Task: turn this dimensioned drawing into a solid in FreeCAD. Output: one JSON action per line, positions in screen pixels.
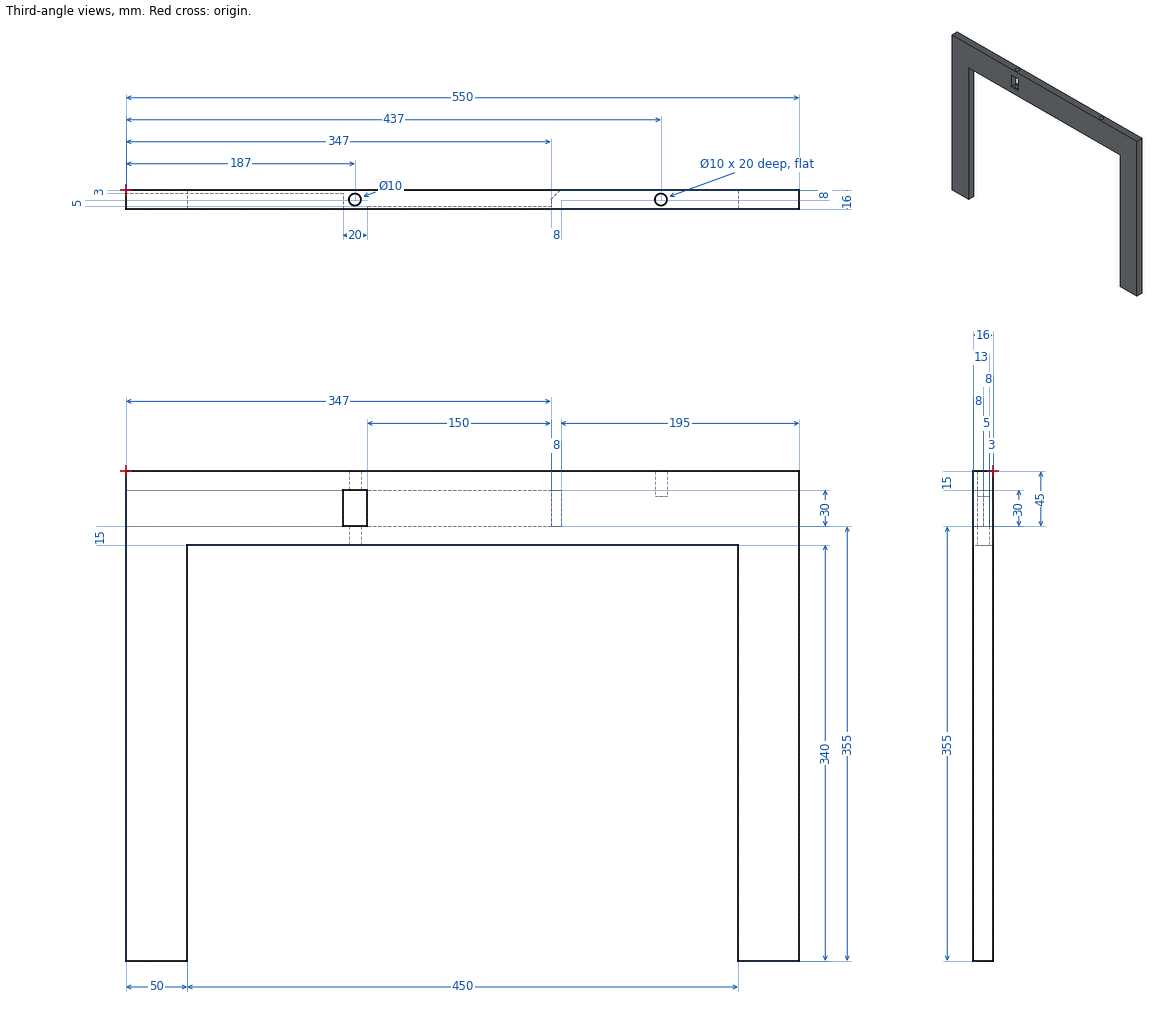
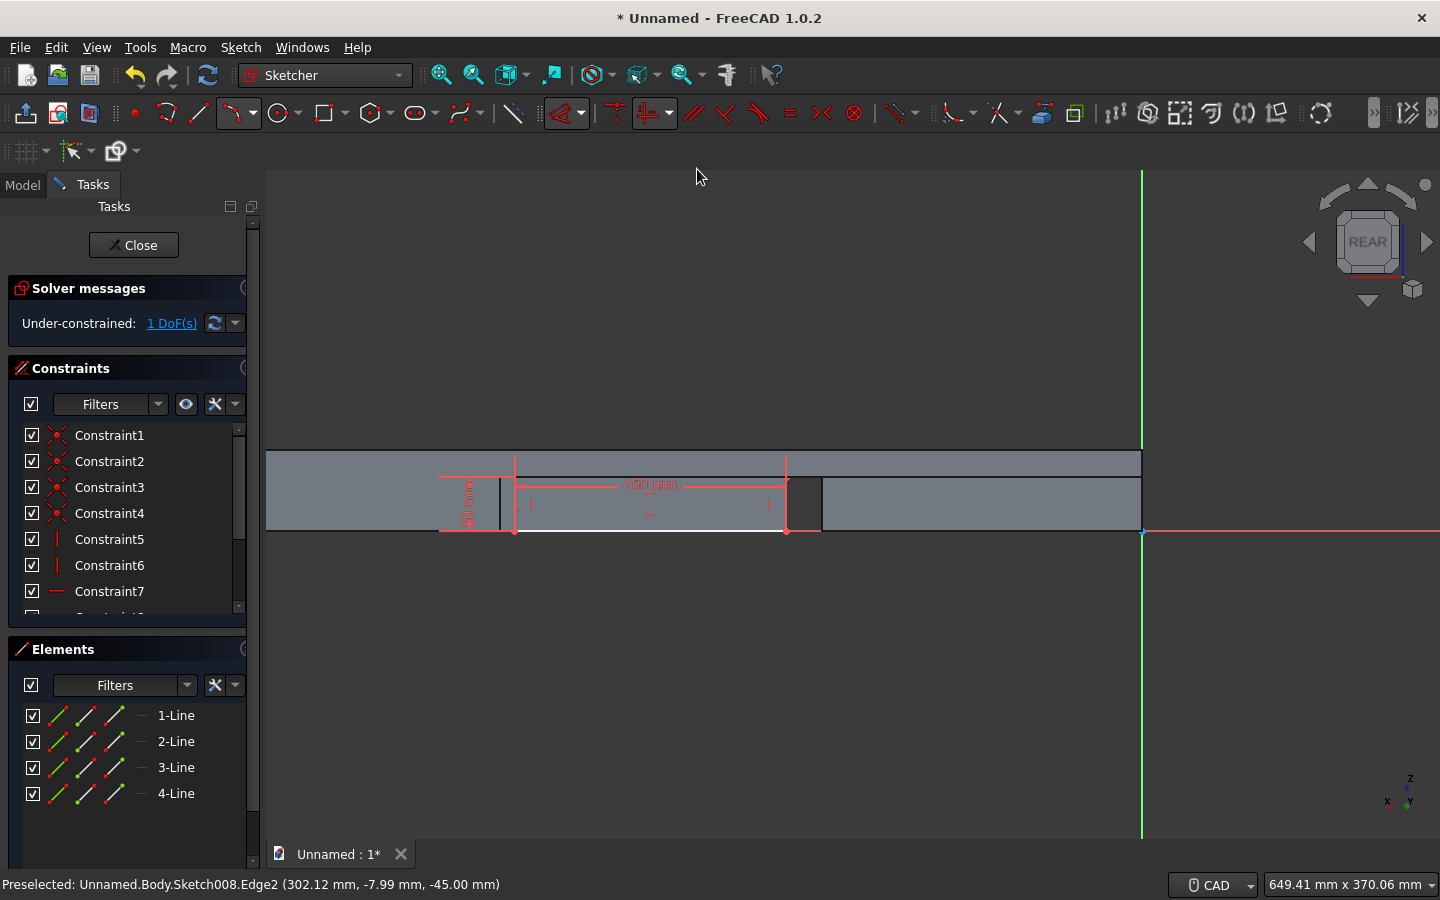
{"action": "left_click", "coordinate": [515, 477]}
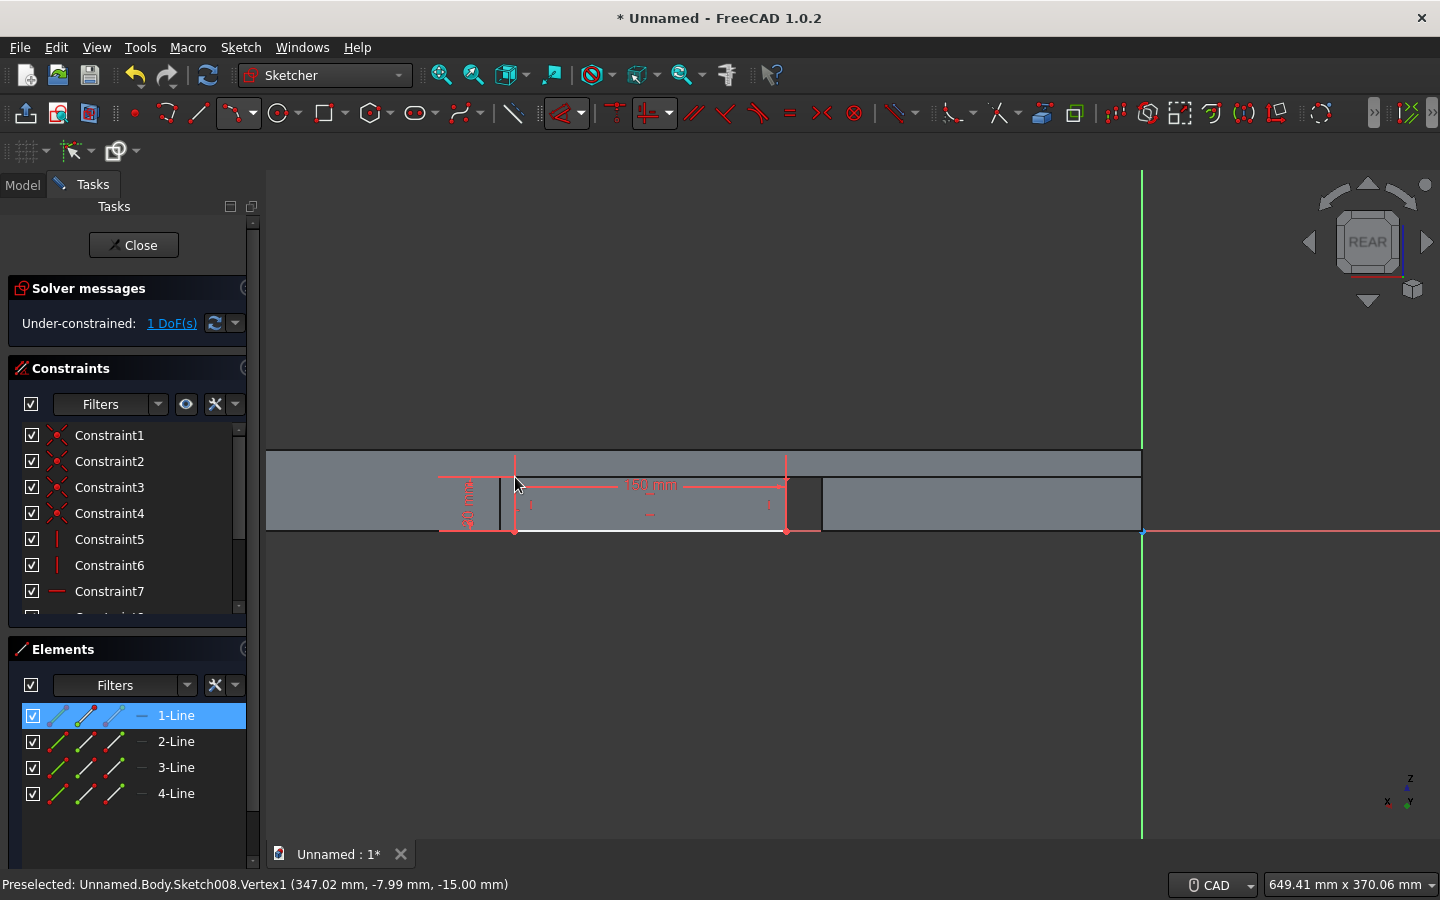
{"action": "key", "text": "l"}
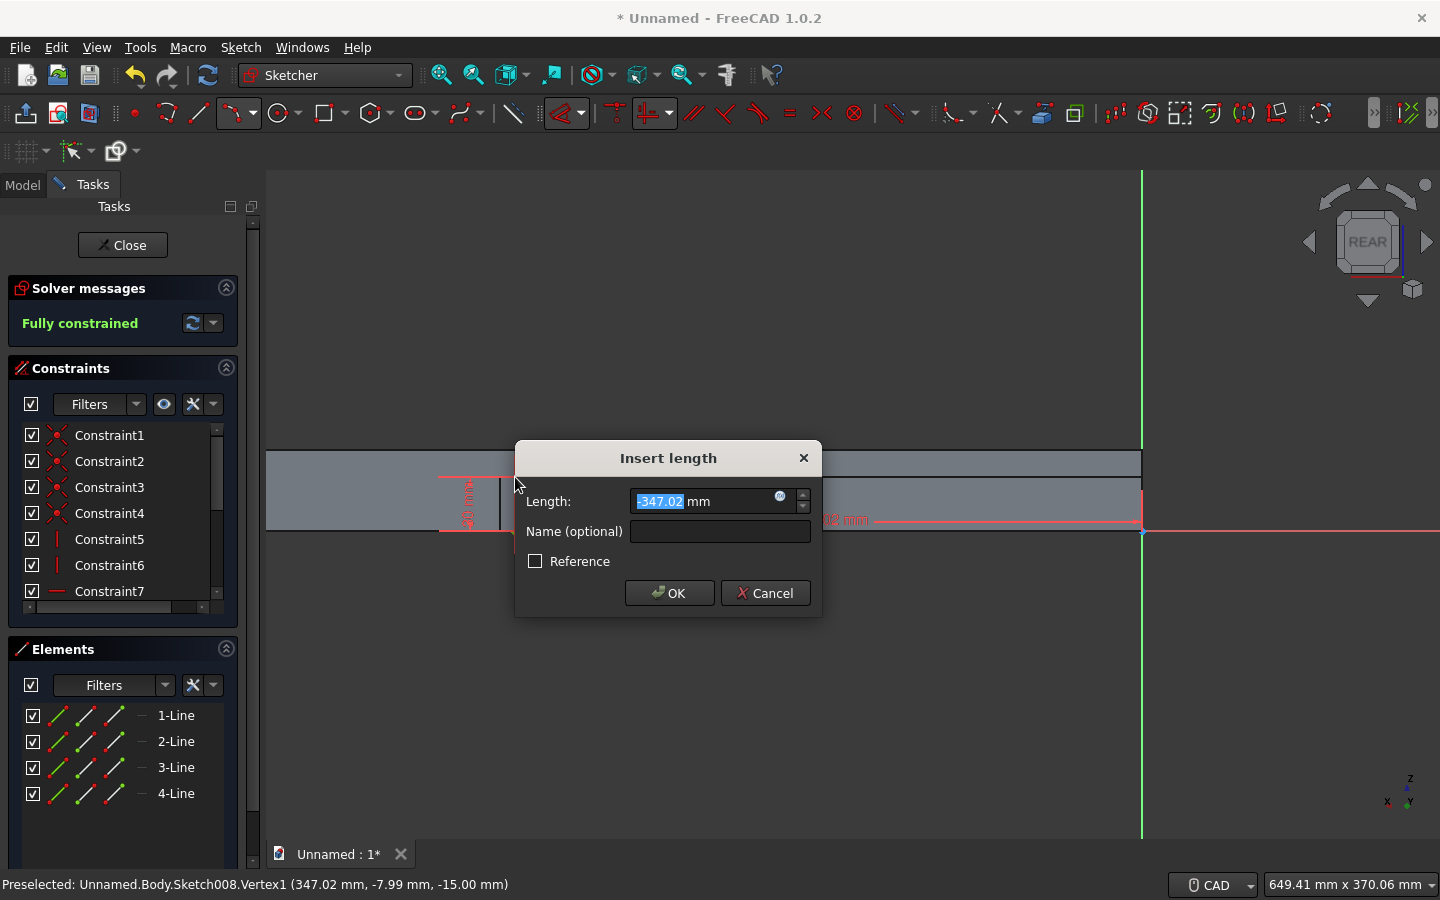
{"action": "type", "text": "-347"}
{"action": "key", "text": "Return"}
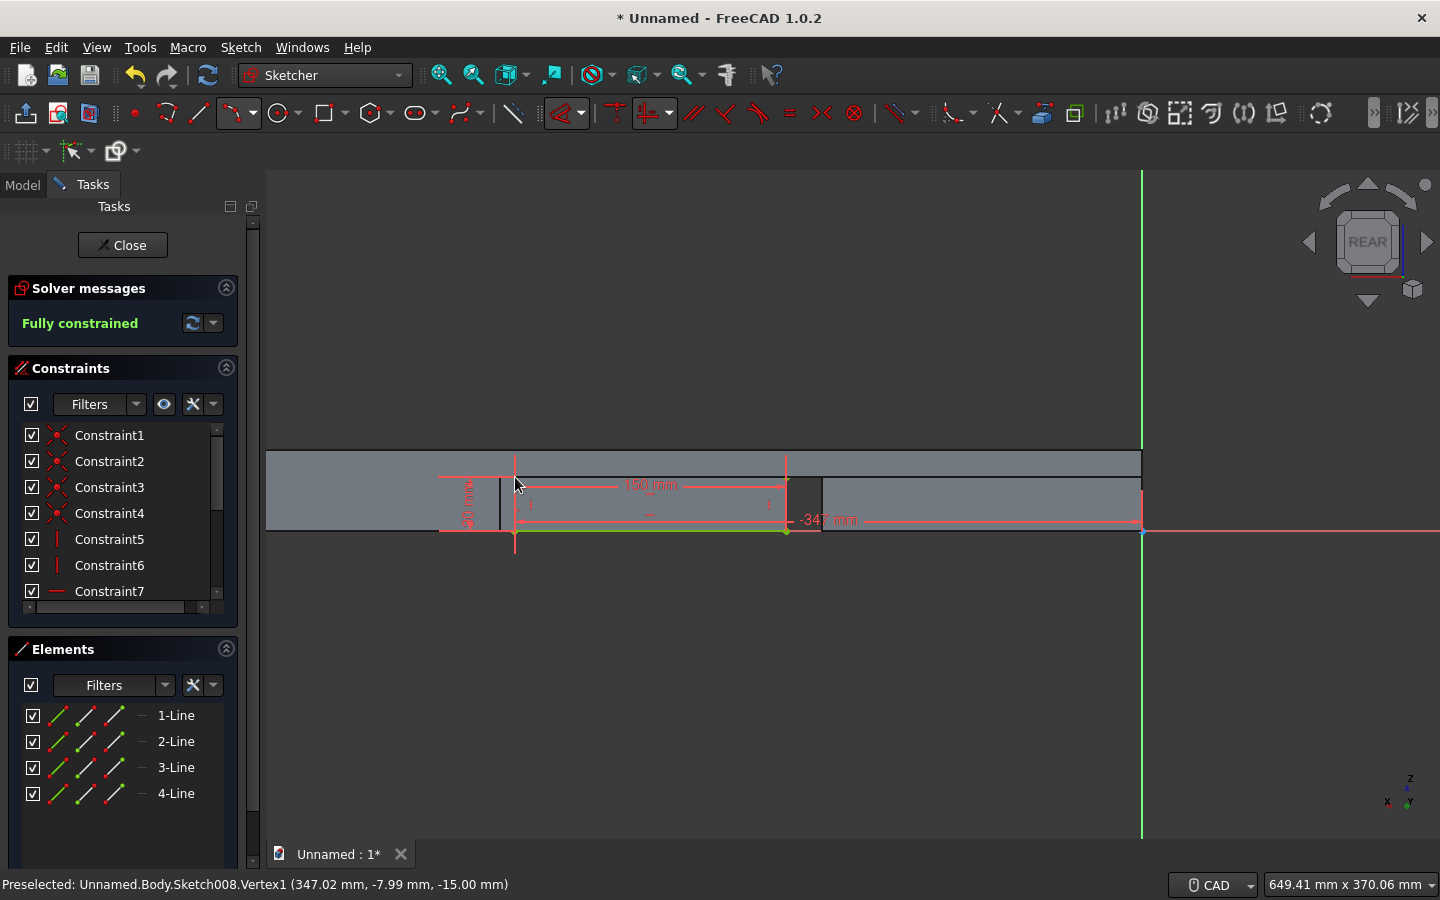
{"action": "left_click", "coordinate": [123, 245]}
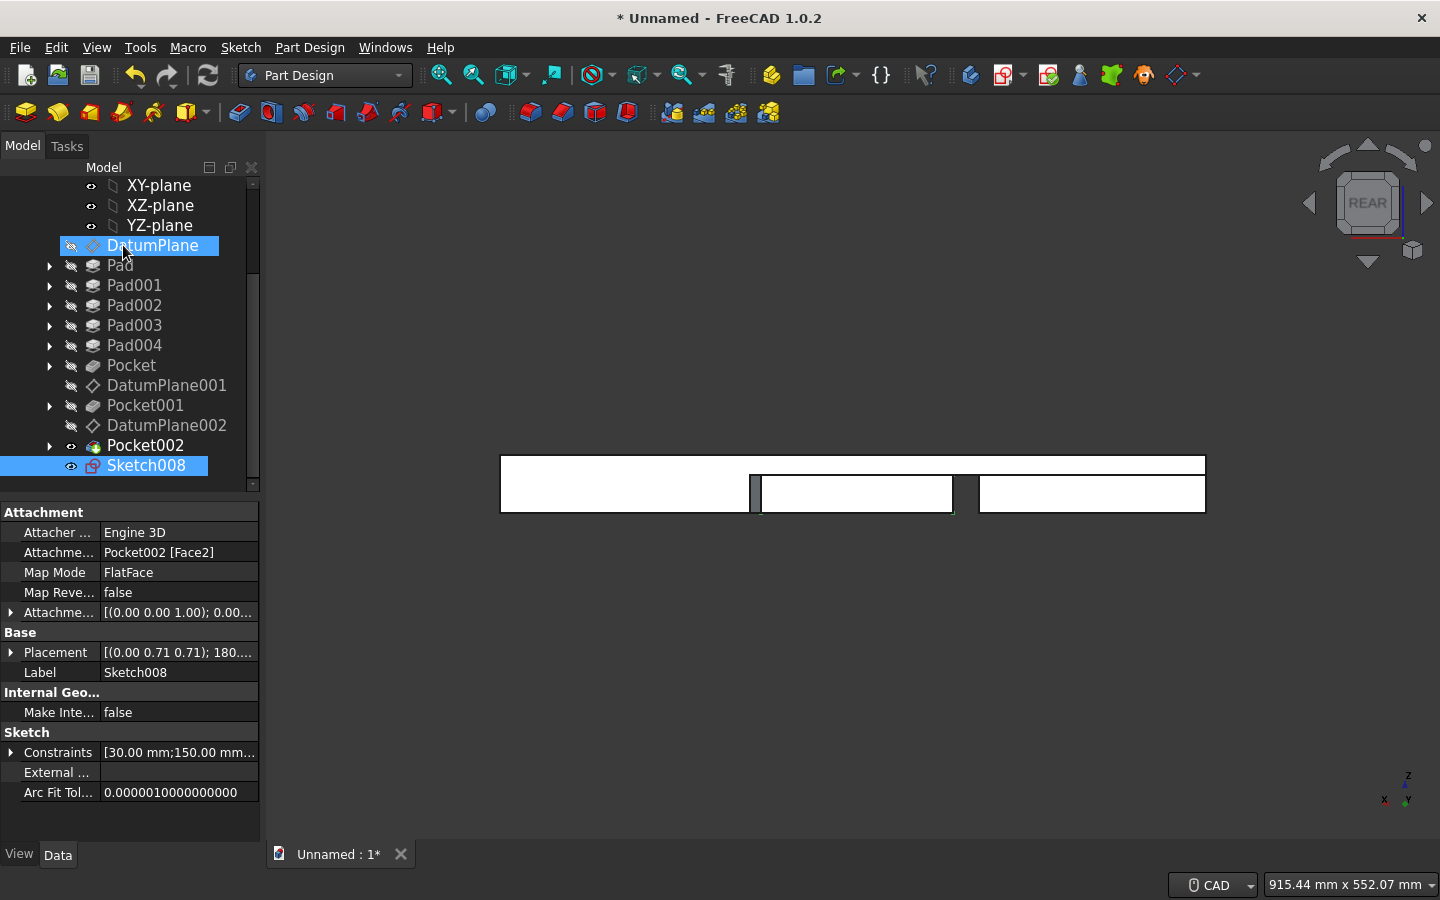
{"action": "left_click", "coordinate": [240, 112]}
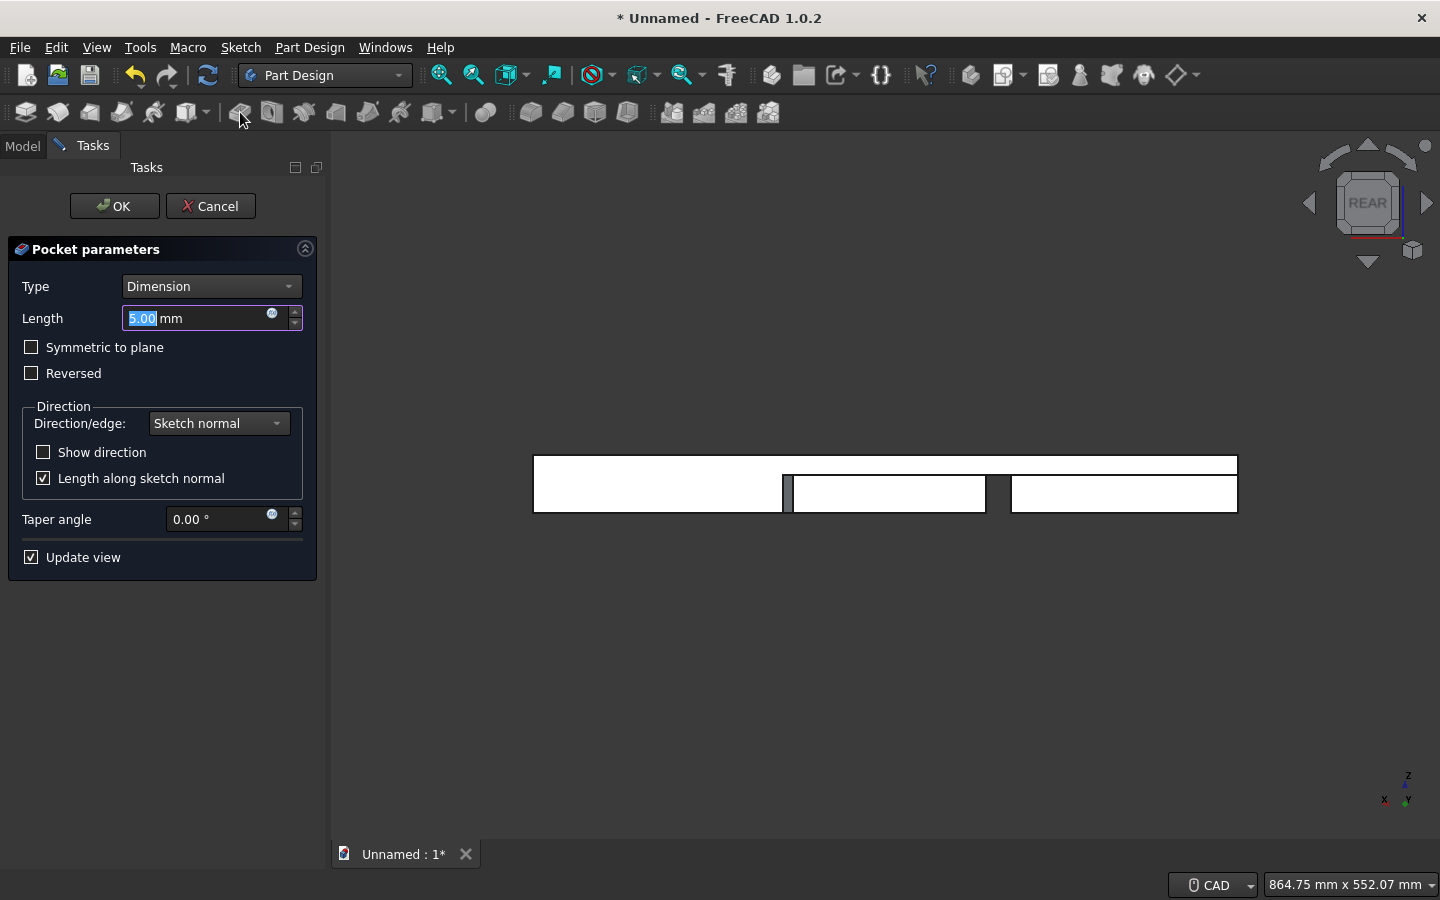
{"action": "type", "text": "5"}
{"action": "key", "text": "Tab"}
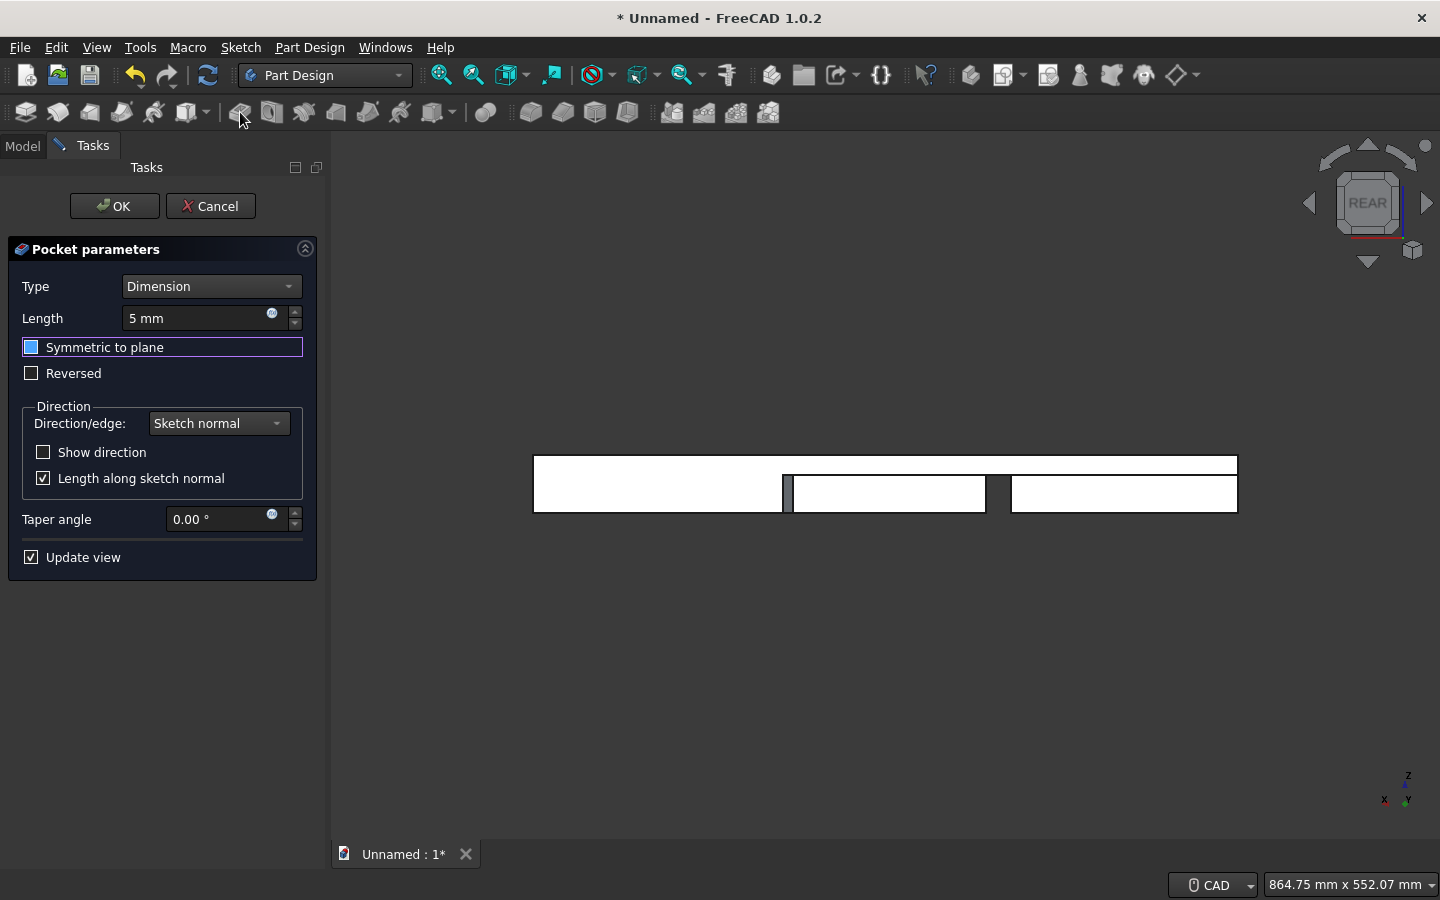
{"action": "left_click", "coordinate": [115, 206]}